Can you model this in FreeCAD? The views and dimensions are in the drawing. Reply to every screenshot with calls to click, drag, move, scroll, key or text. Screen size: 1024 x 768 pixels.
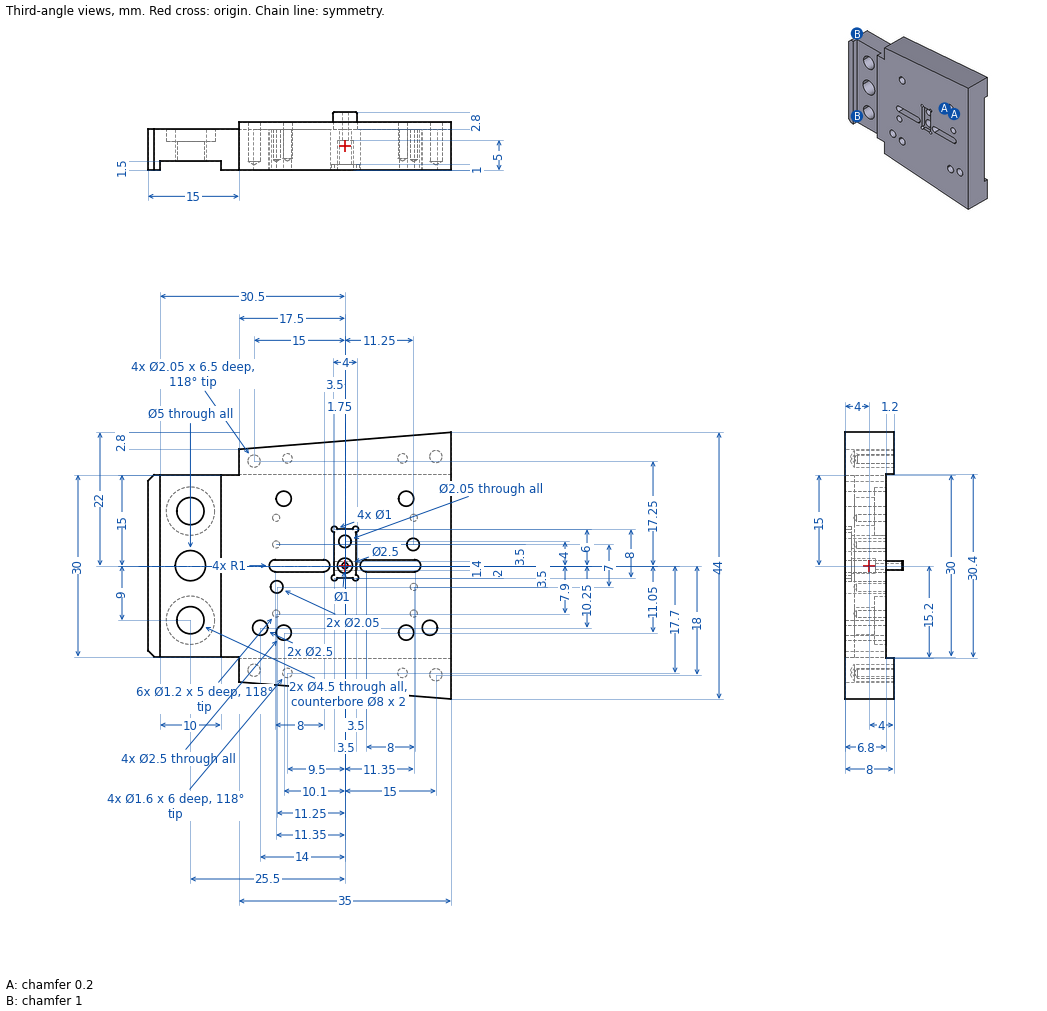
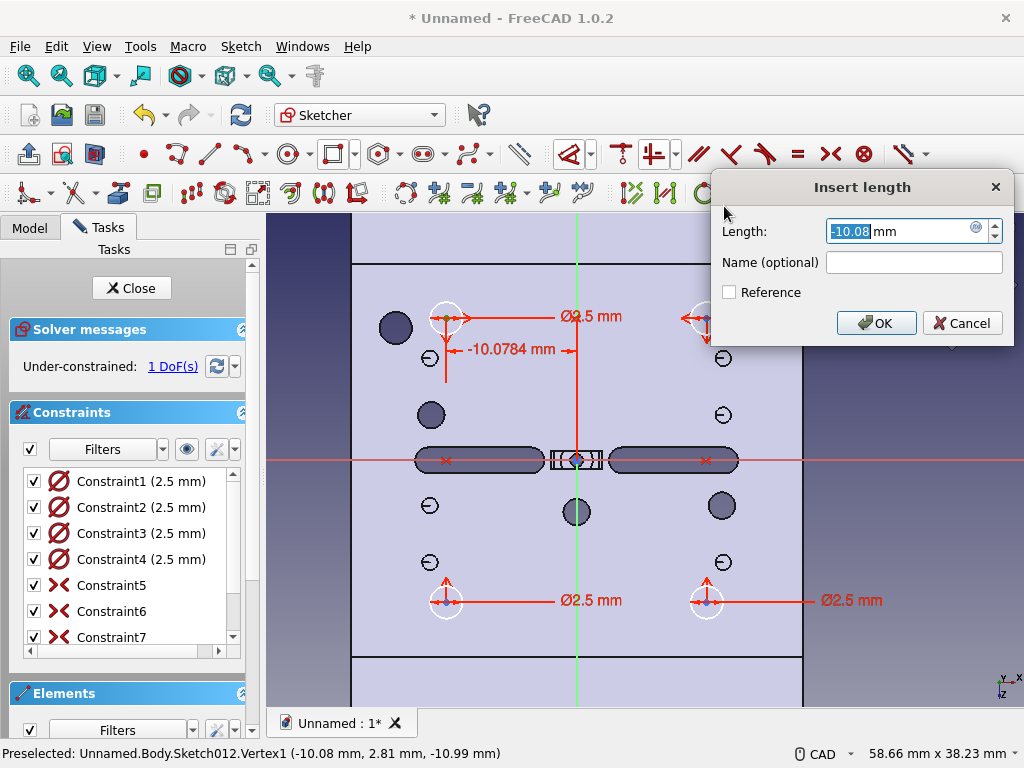
text(-10.1)
key(Return)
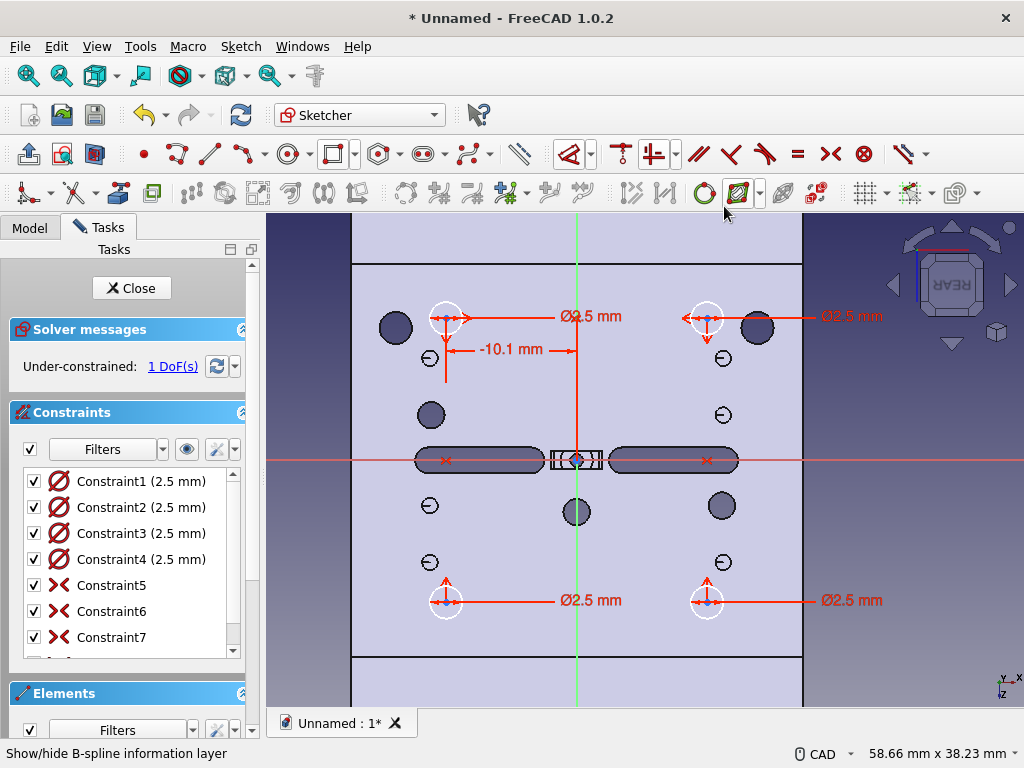
click(446, 318)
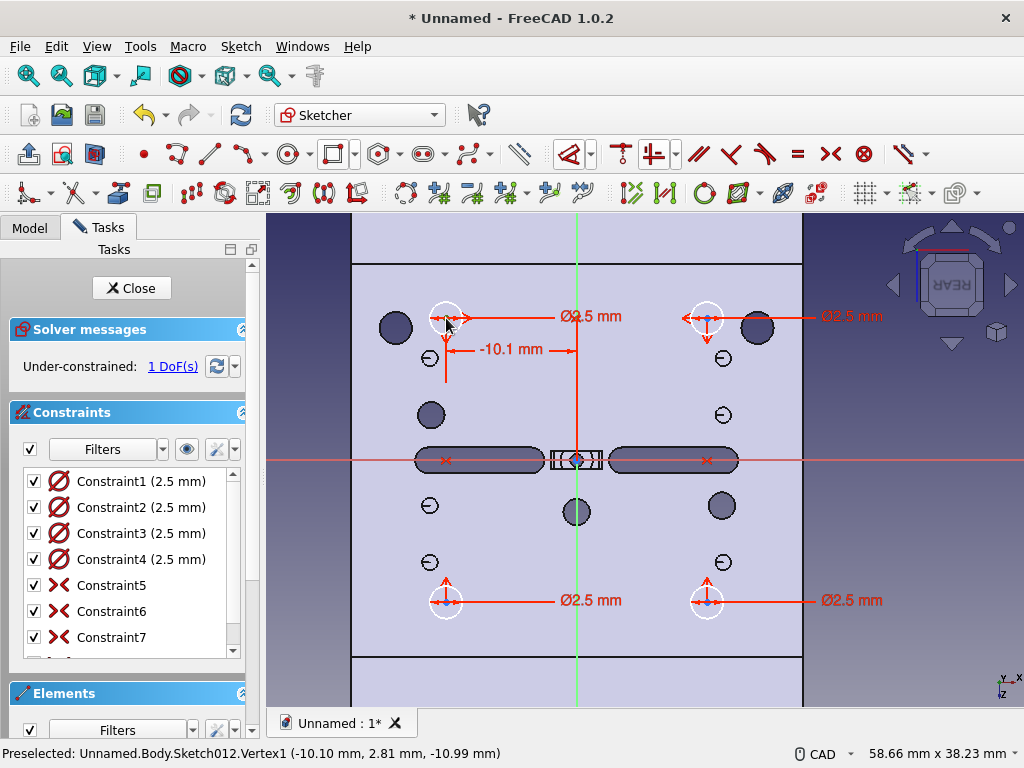
click(590, 154)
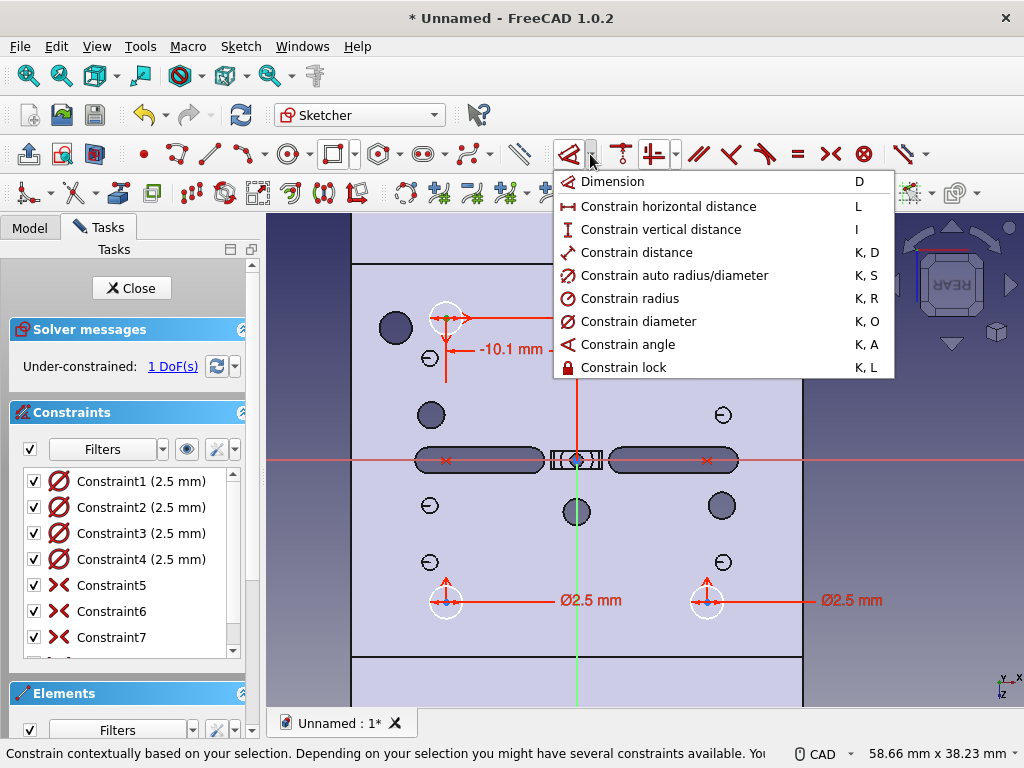
click(724, 230)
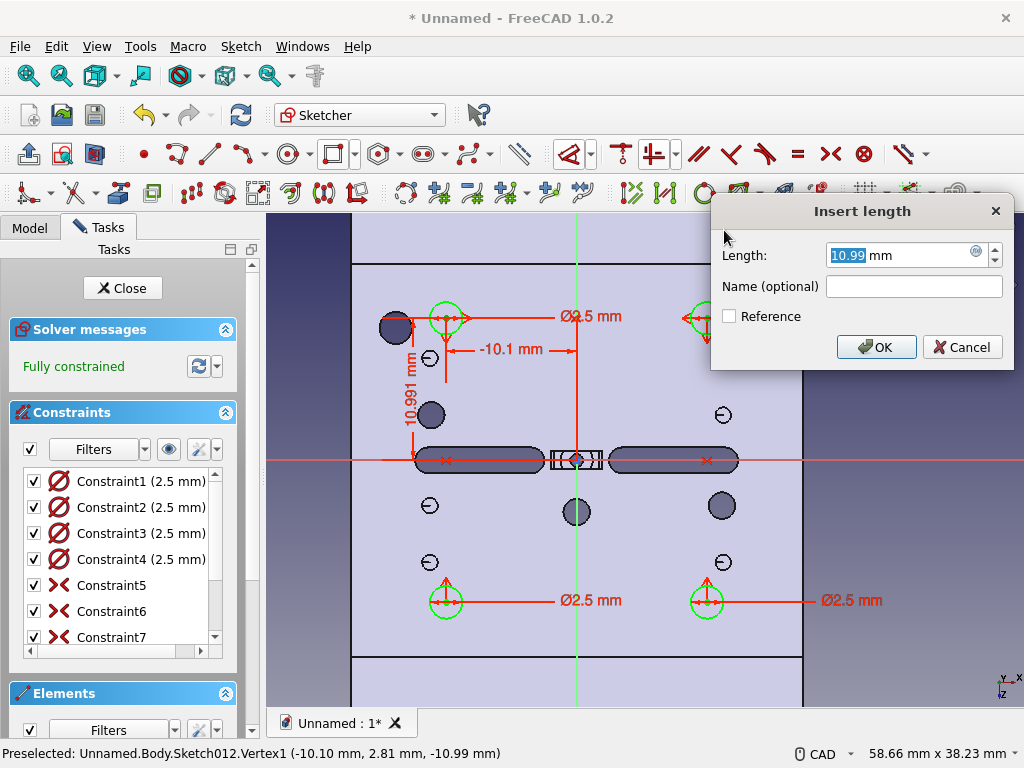
text(11.05)
key(Return)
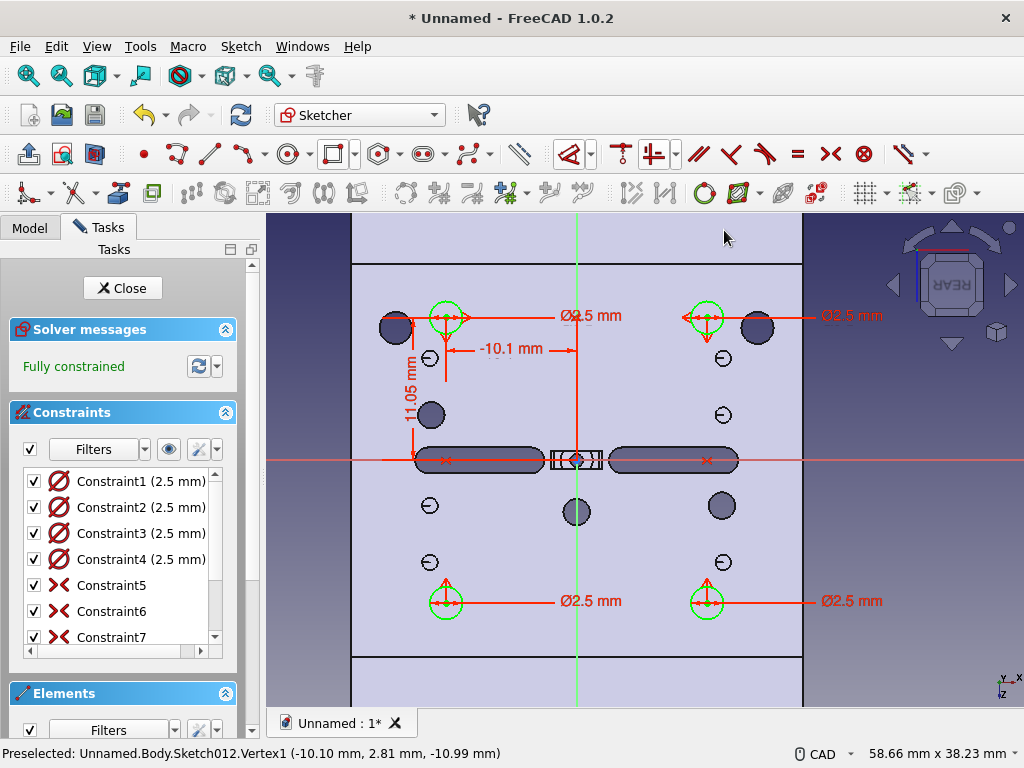
click(123, 288)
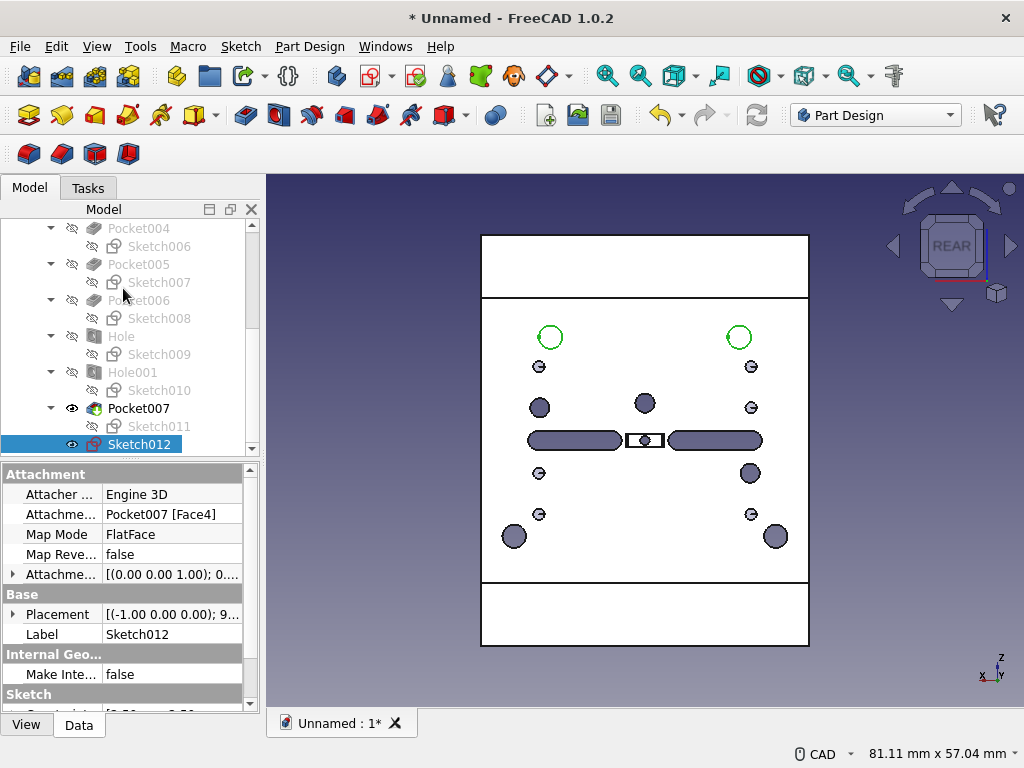
click(279, 116)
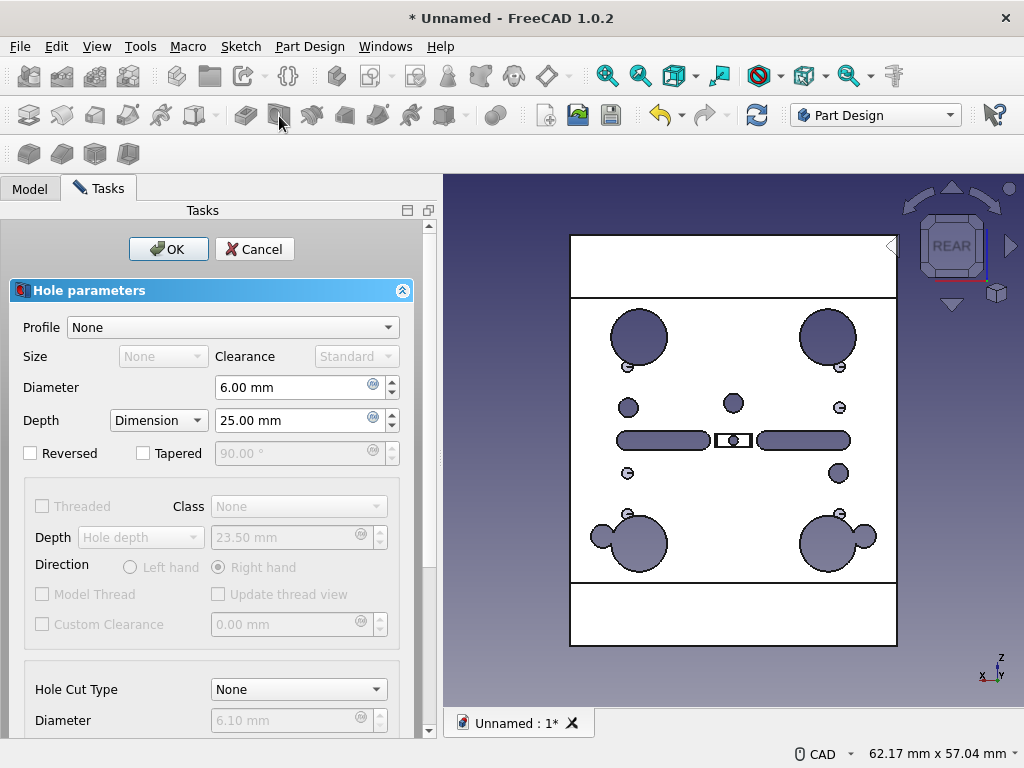
triple_click(300, 388)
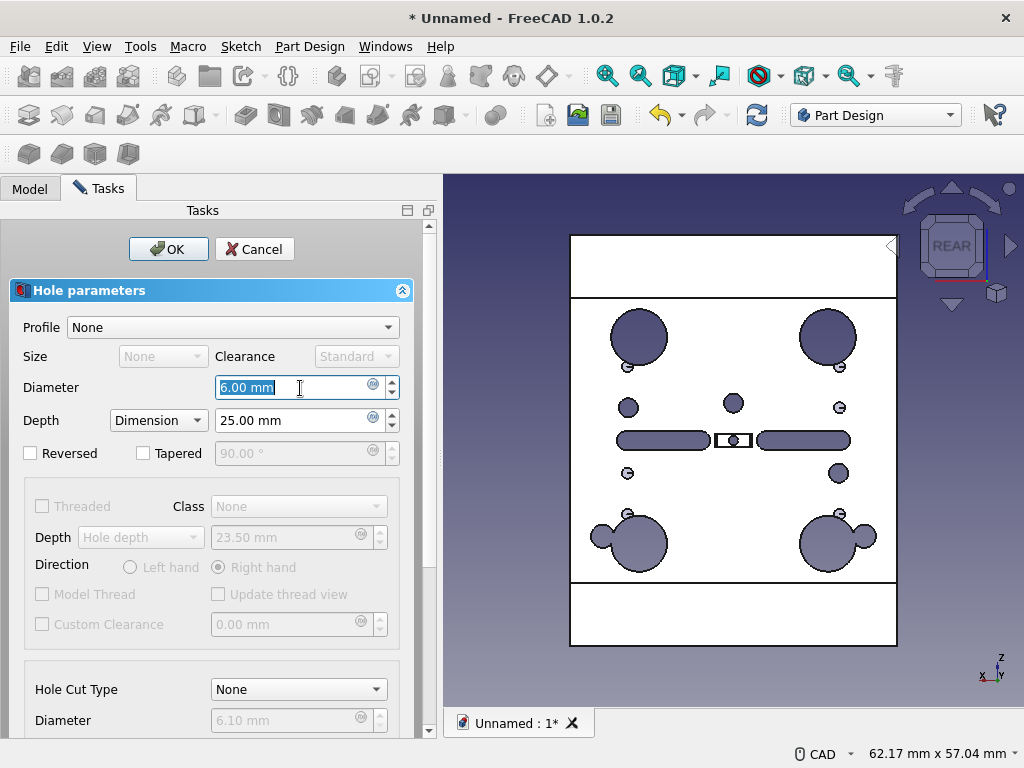
text(2.5)
key(Tab)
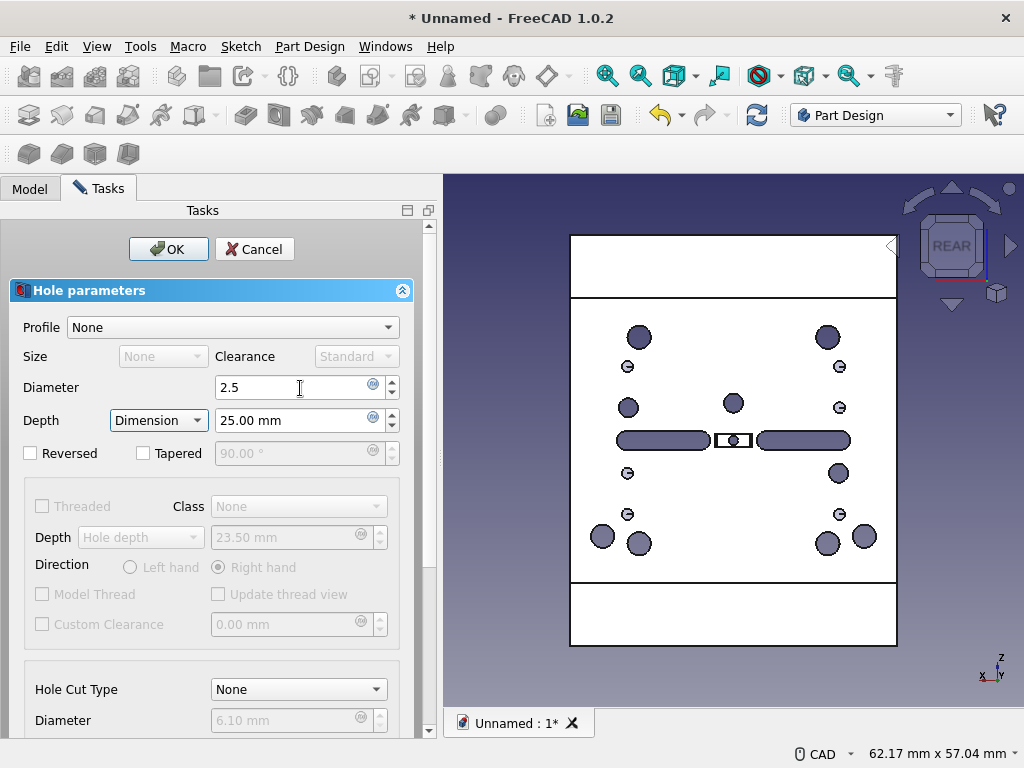
click(160, 420)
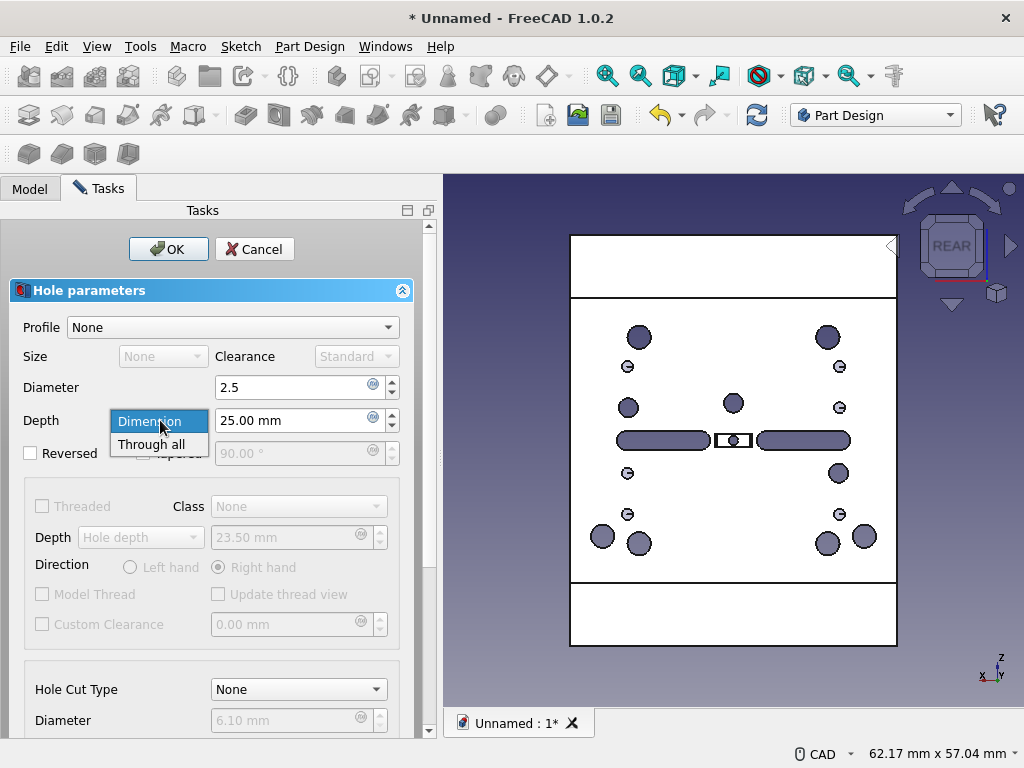
click(158, 444)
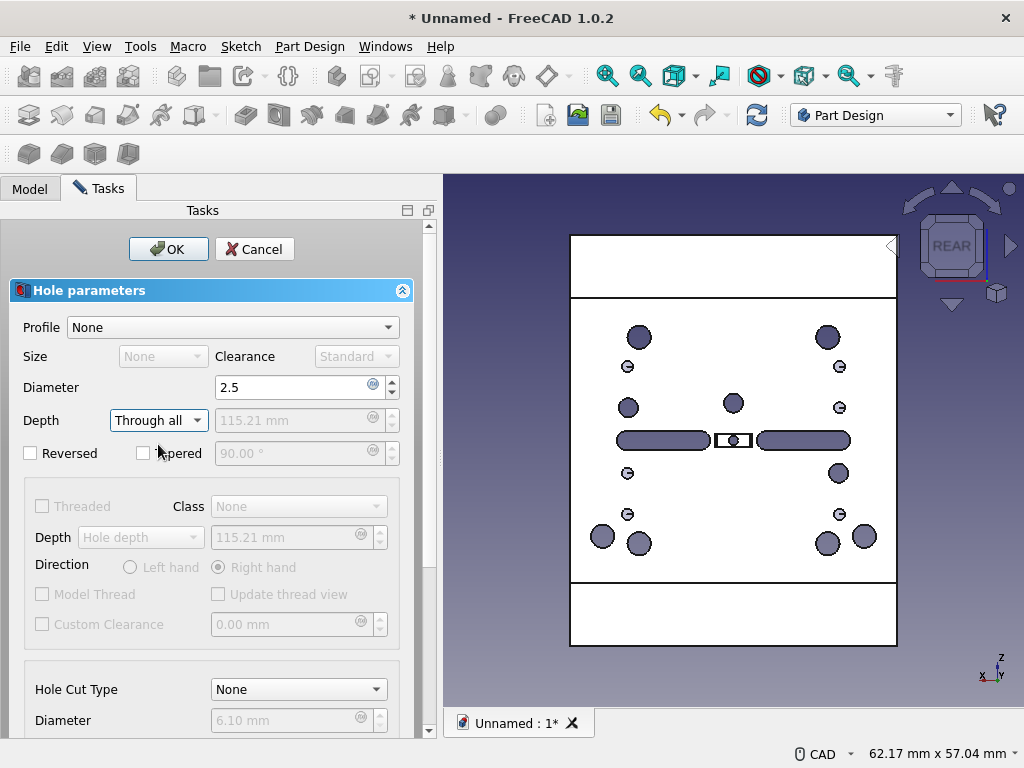
click(169, 249)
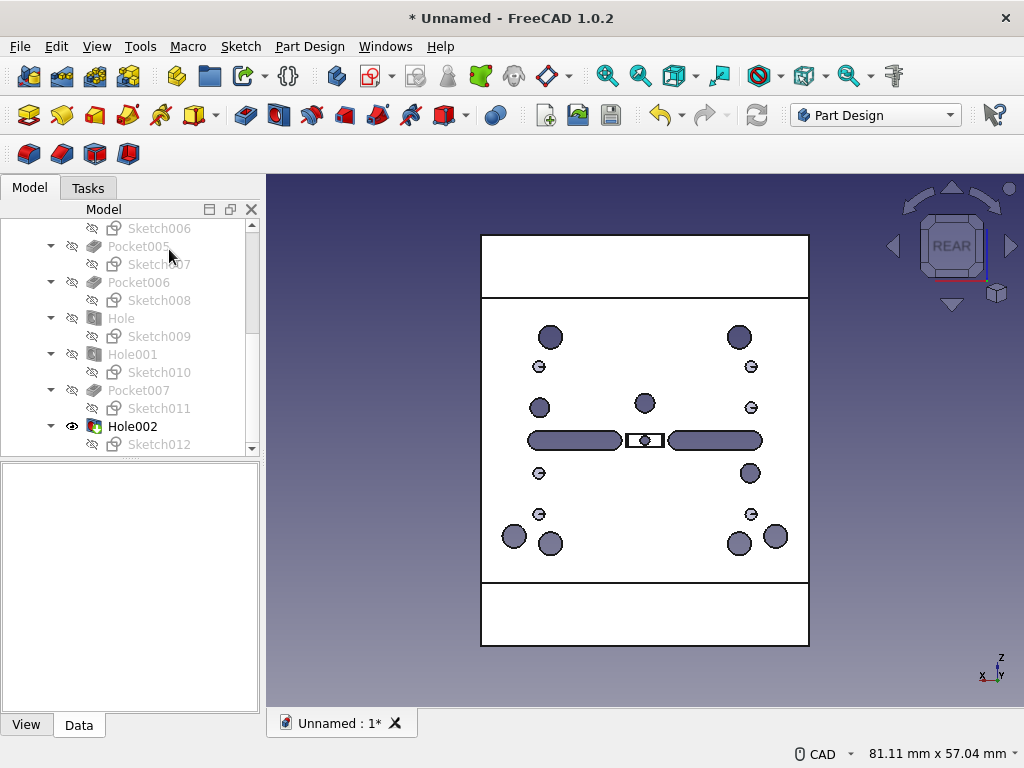
click(692, 613)